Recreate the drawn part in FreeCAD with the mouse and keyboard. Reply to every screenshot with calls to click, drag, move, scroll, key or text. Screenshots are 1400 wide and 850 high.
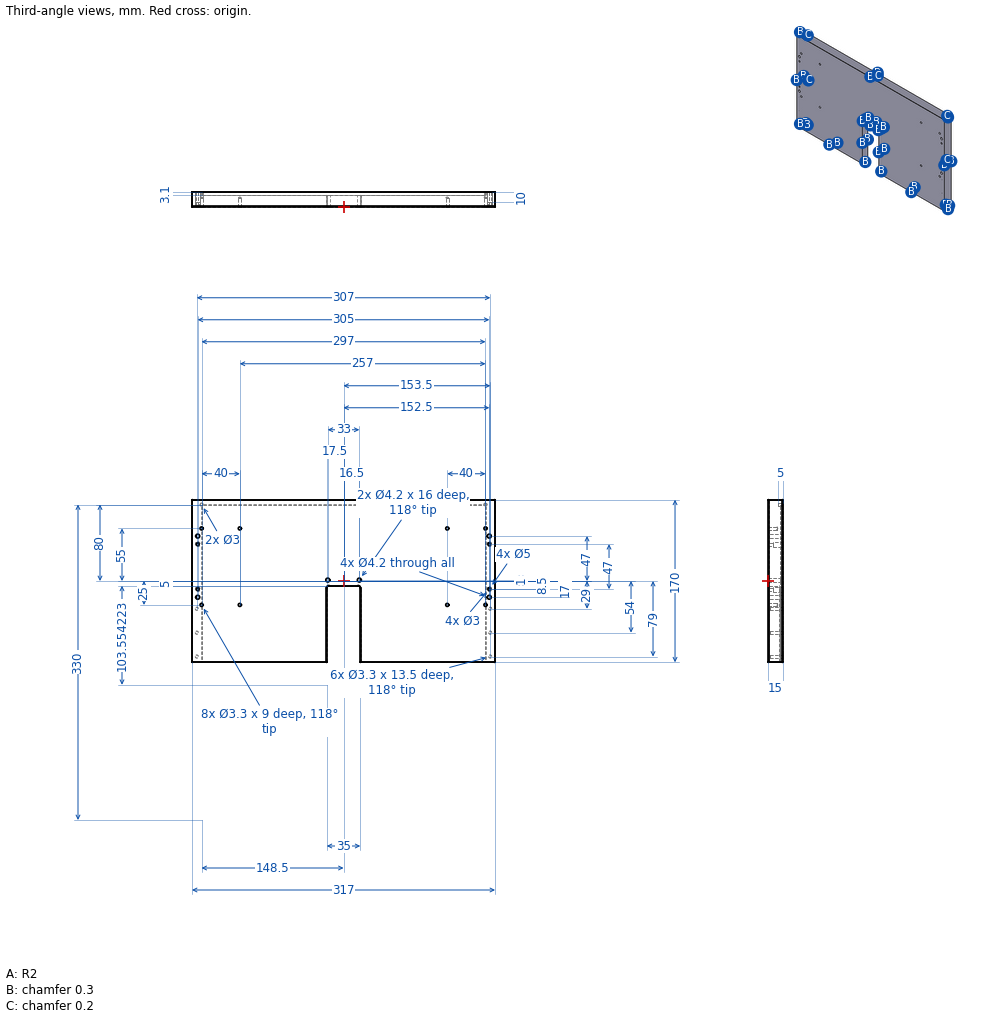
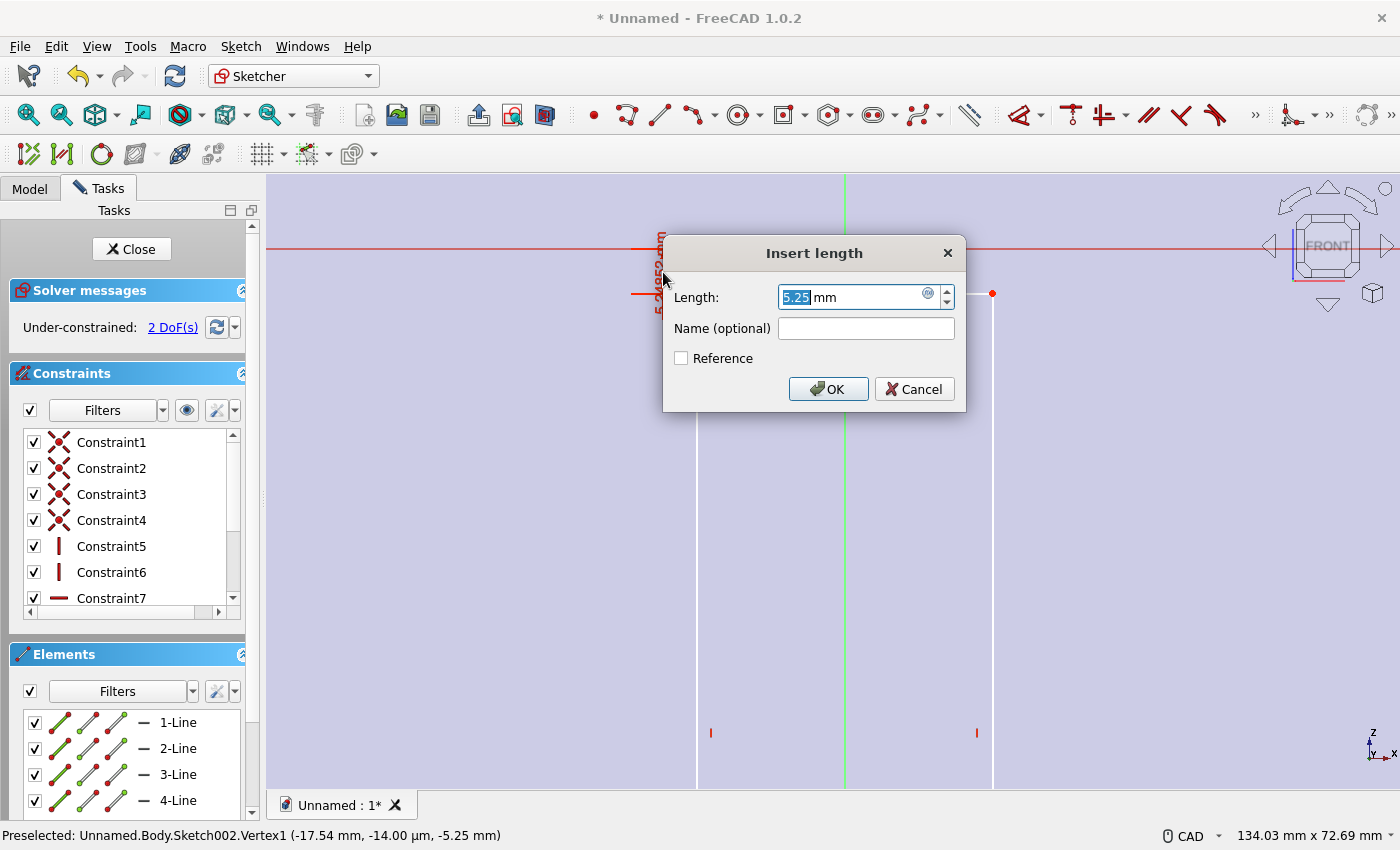
text(5)
key(Return)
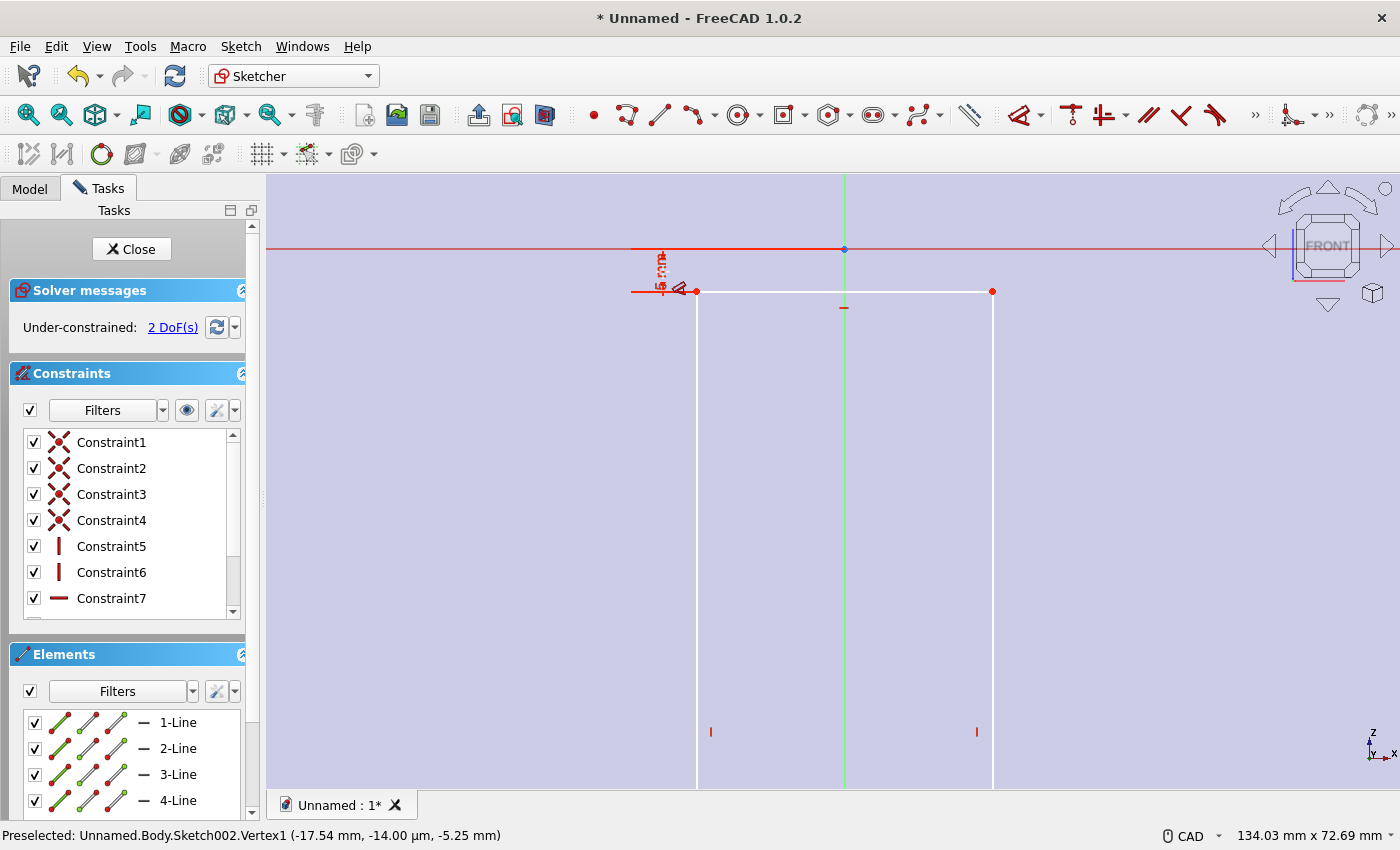
click(697, 292)
click(771, 215)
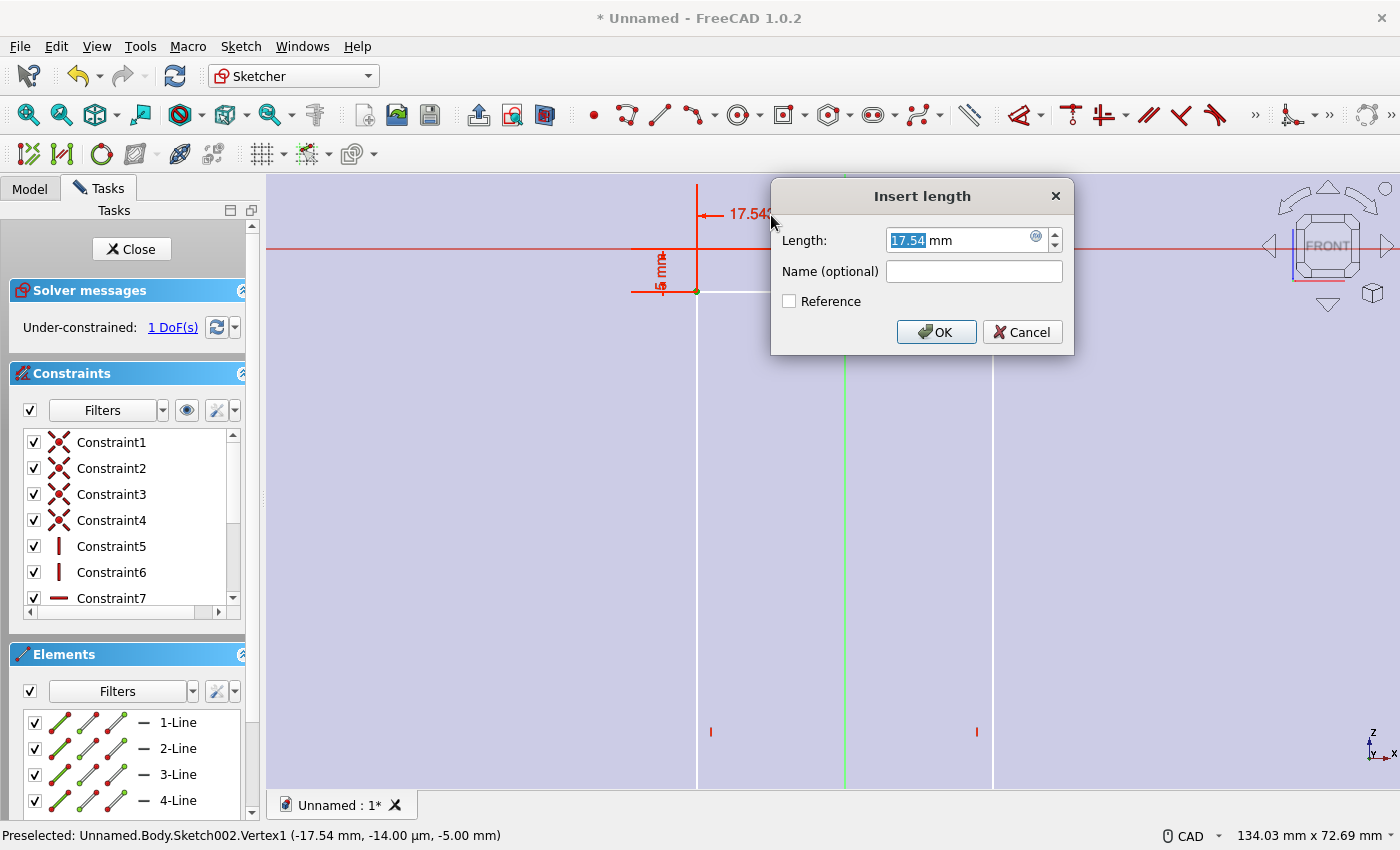
text(17.5)
key(Return)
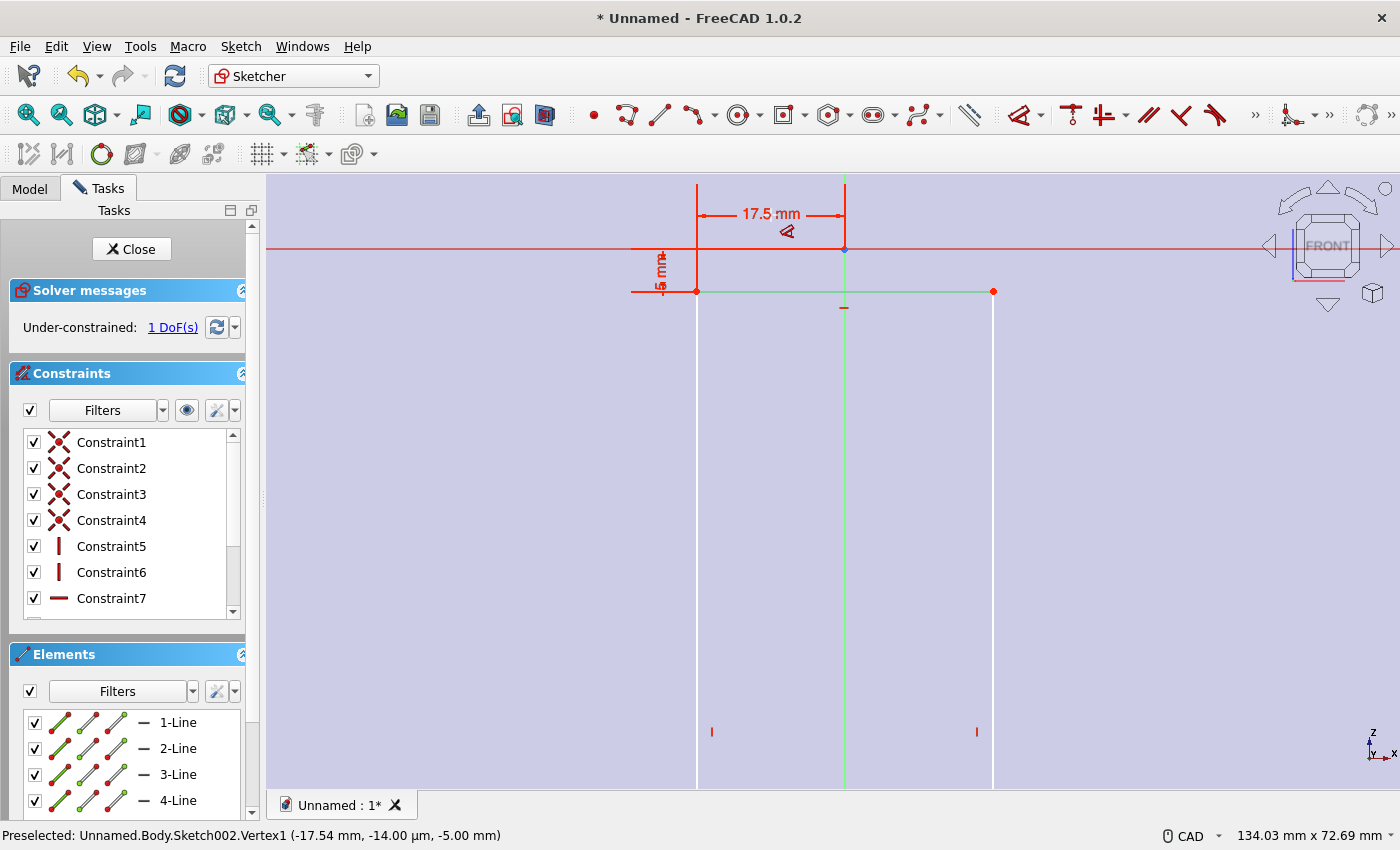
click(697, 555)
click(663, 526)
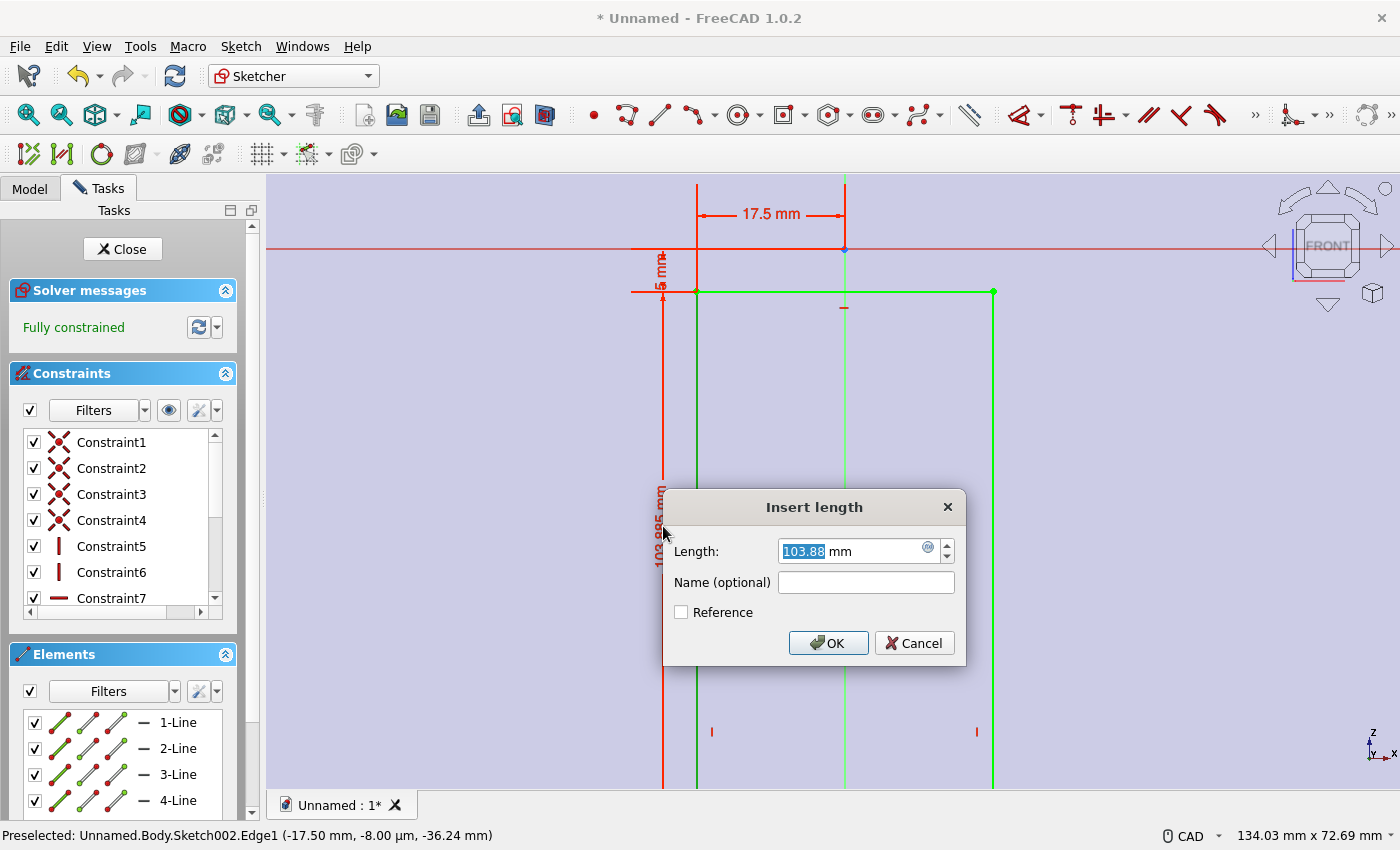
text(103.554223)
key(Return)
key(Escape)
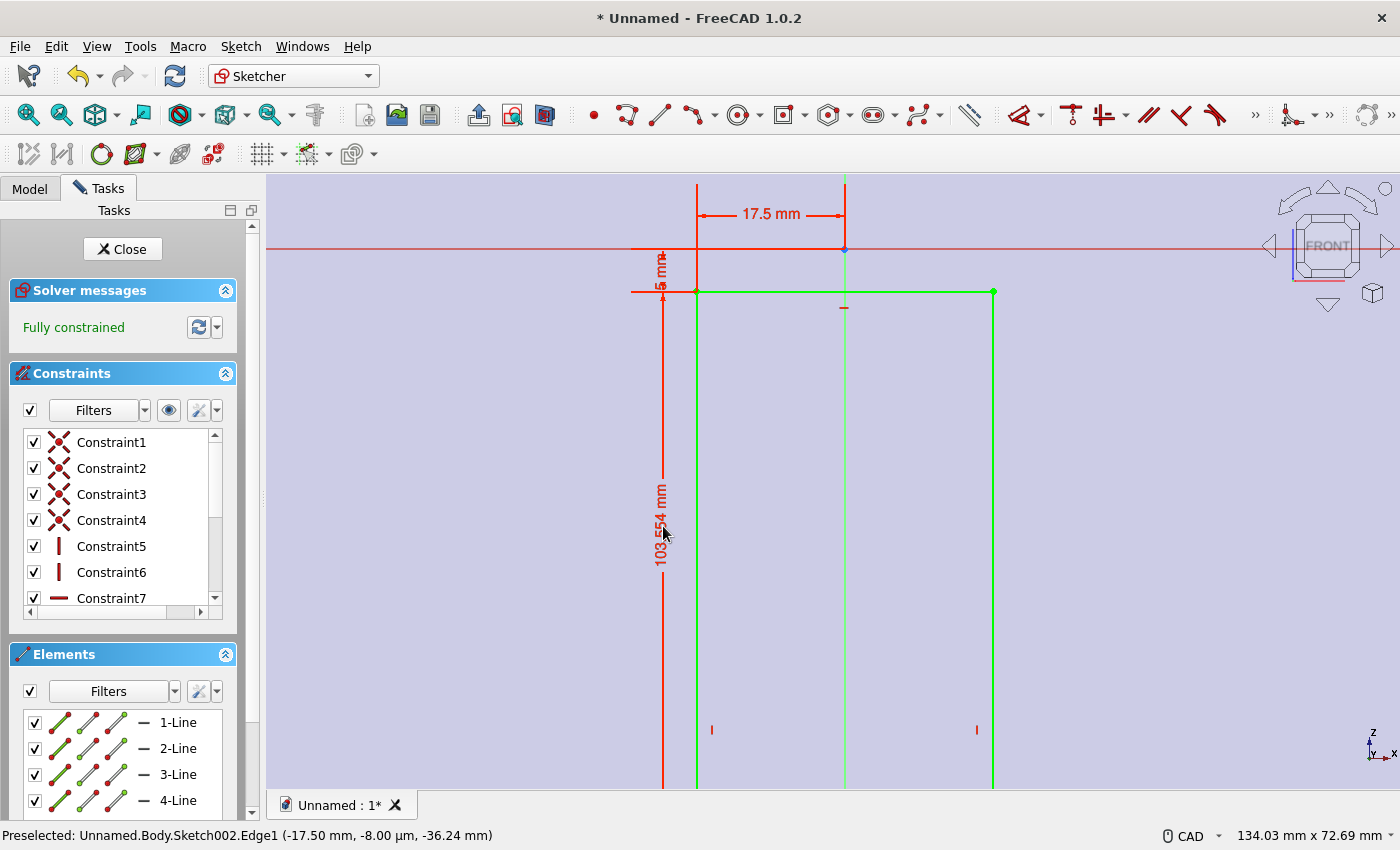
click(123, 249)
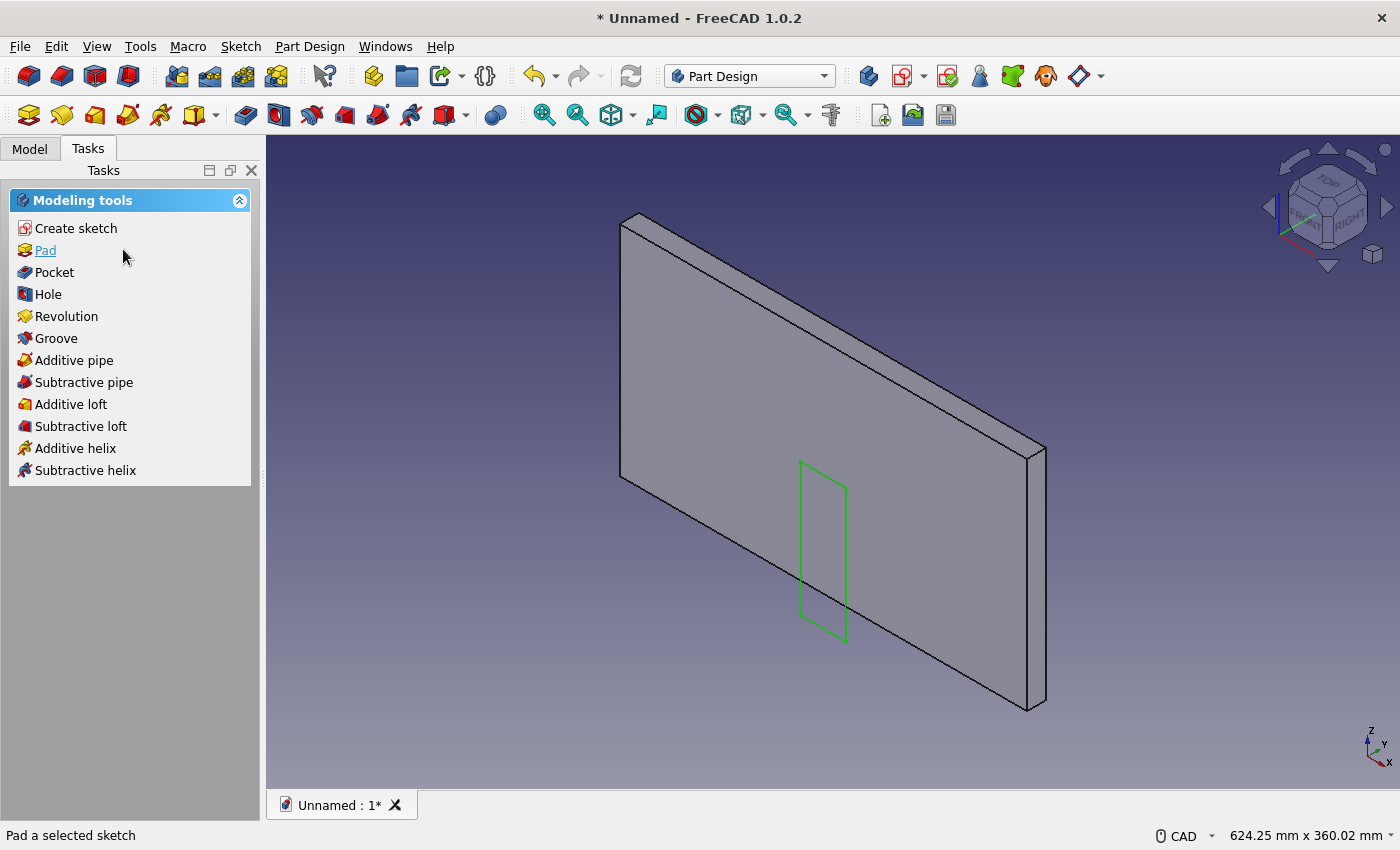
click(246, 116)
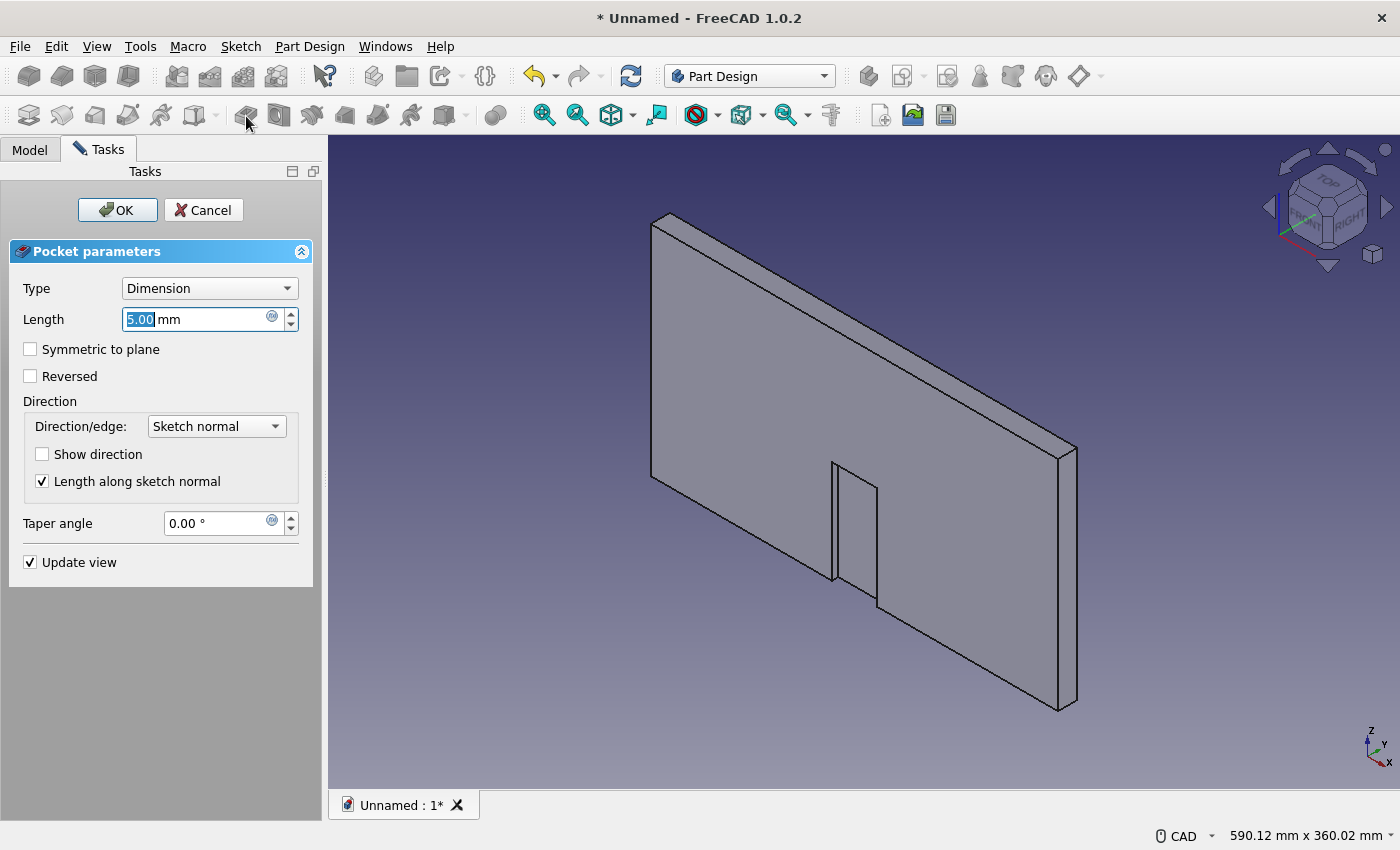
click(210, 288)